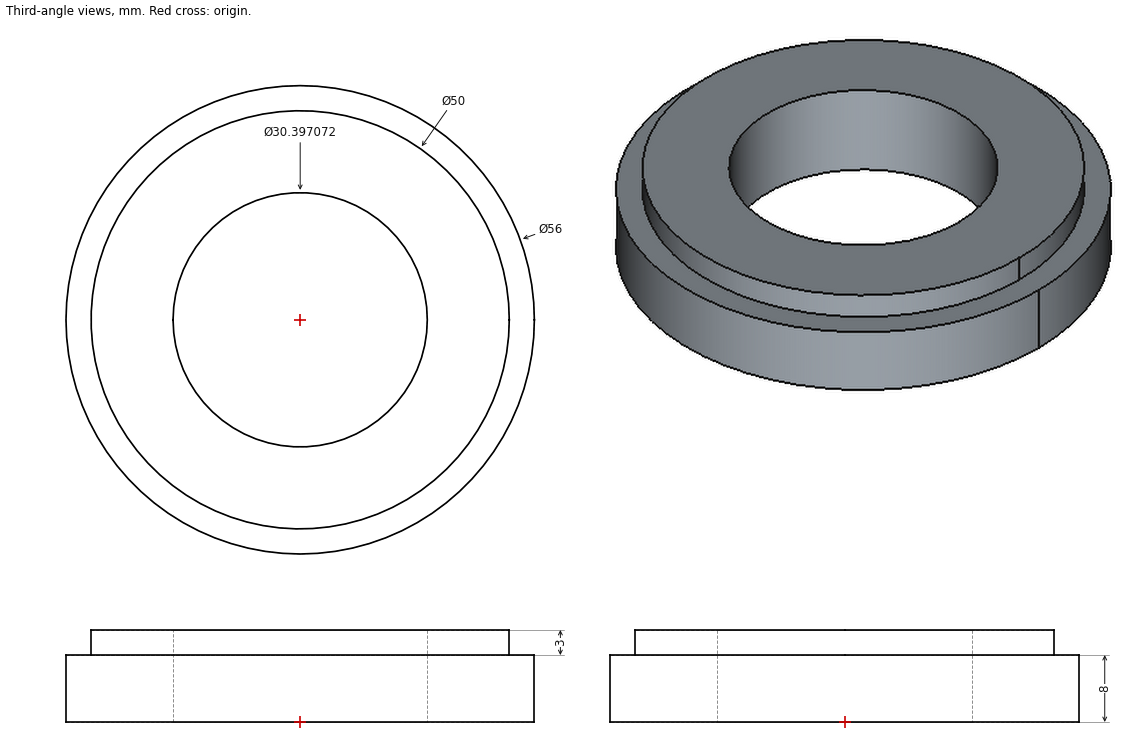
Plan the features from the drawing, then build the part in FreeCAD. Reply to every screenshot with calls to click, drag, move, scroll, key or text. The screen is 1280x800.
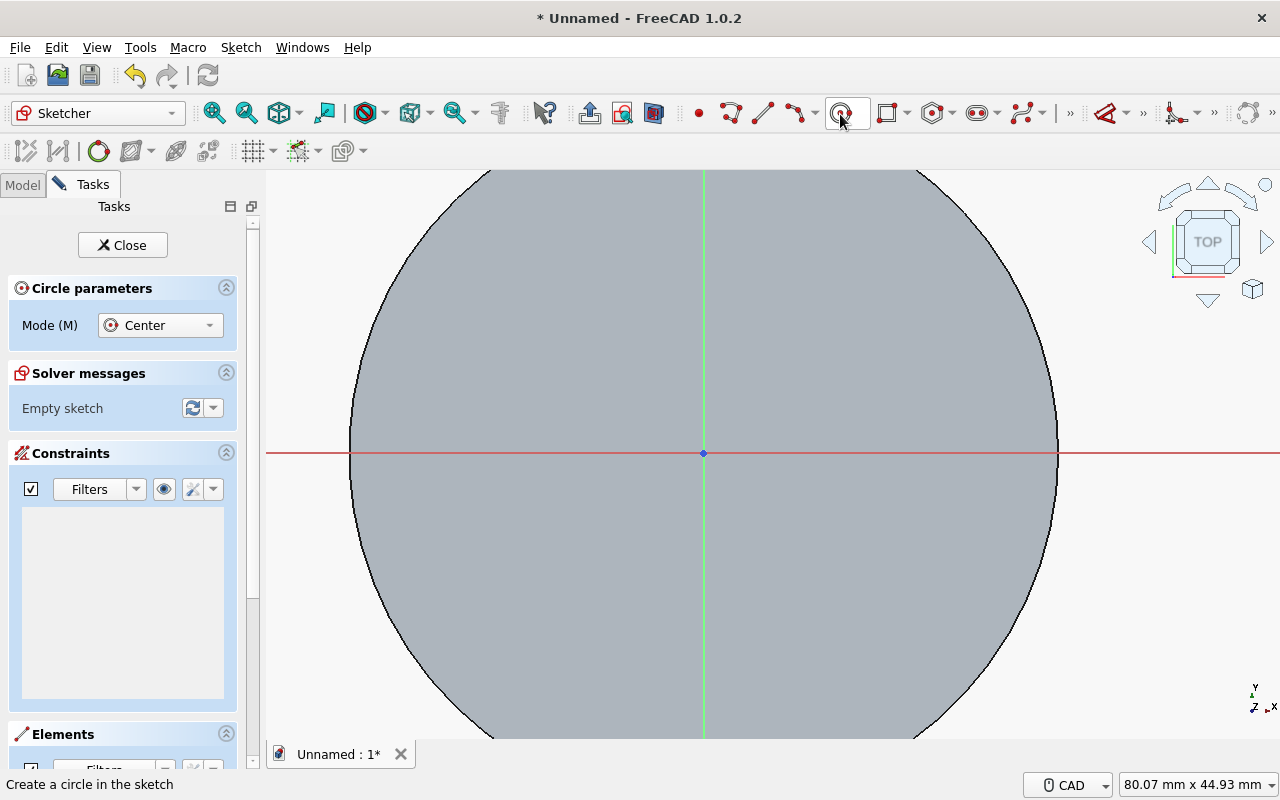
click(704, 453)
click(840, 317)
key(Escape)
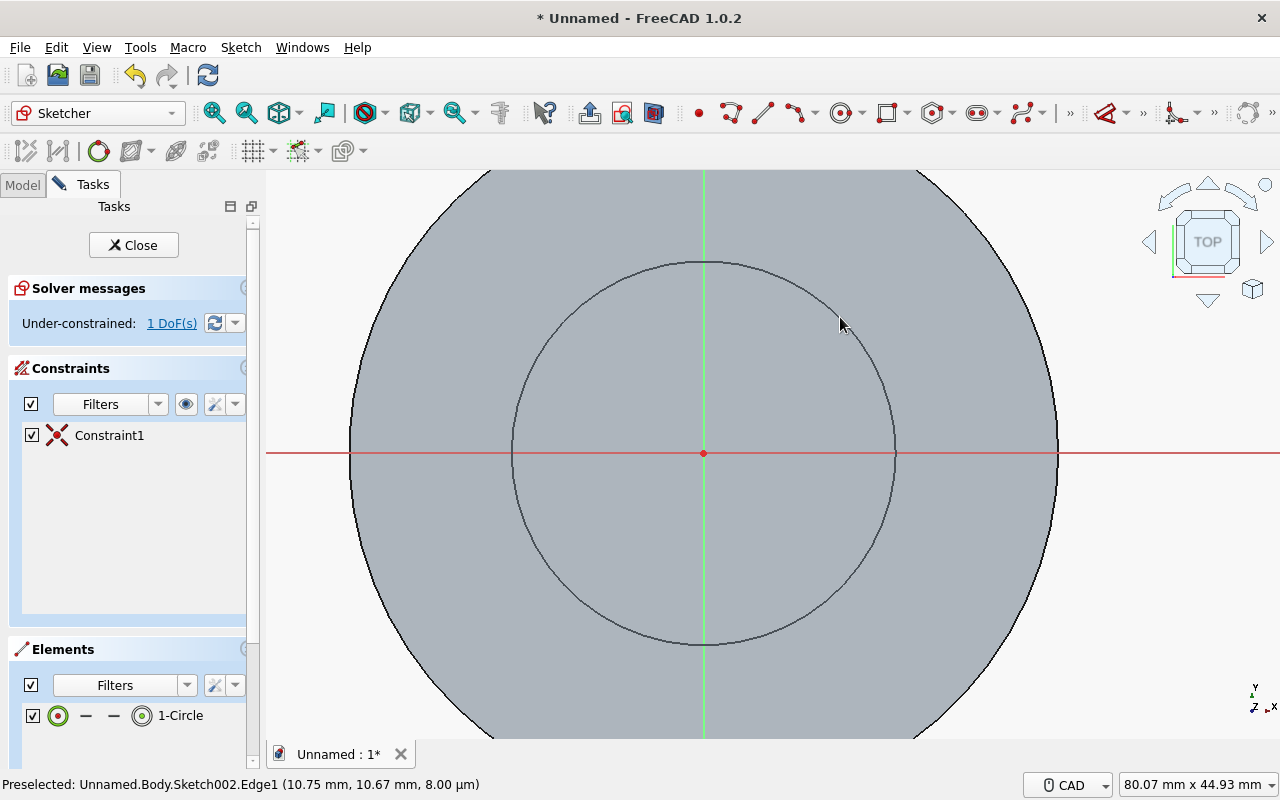
click(1106, 114)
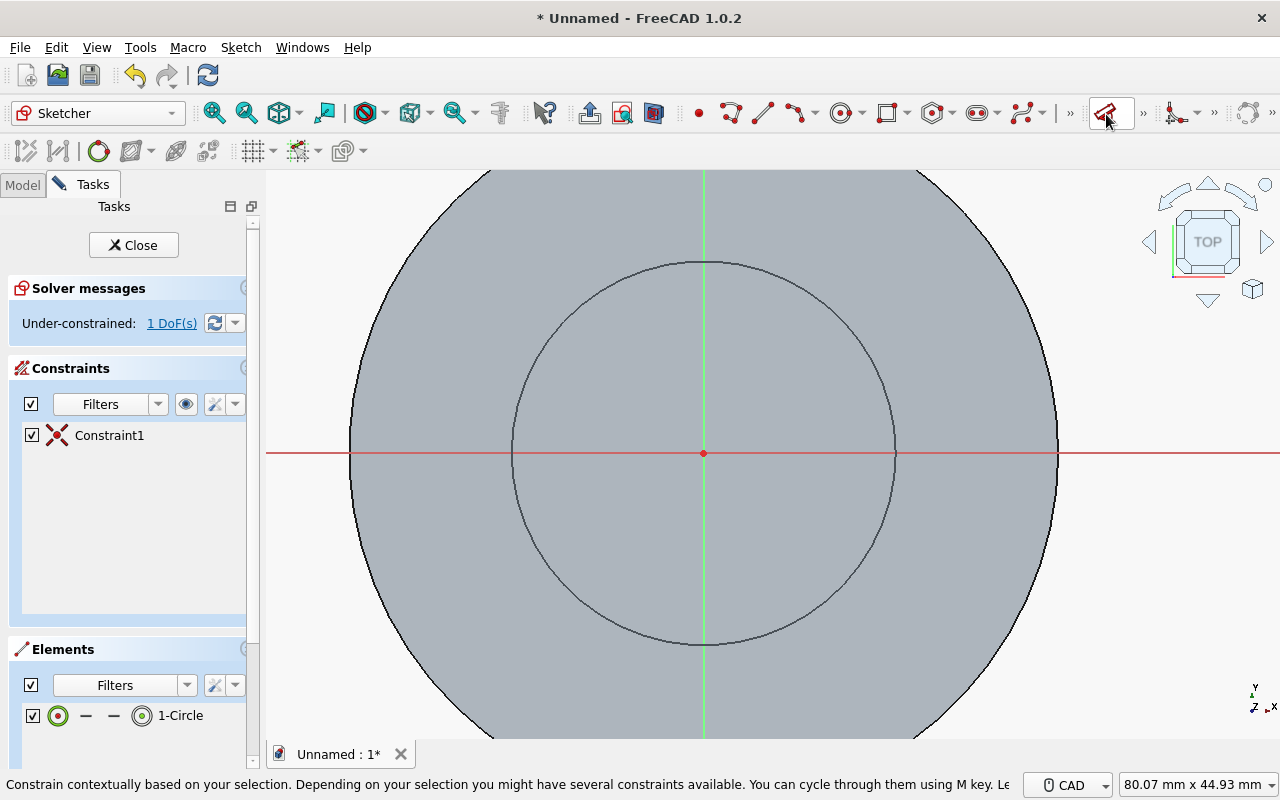
click(839, 317)
click(862, 294)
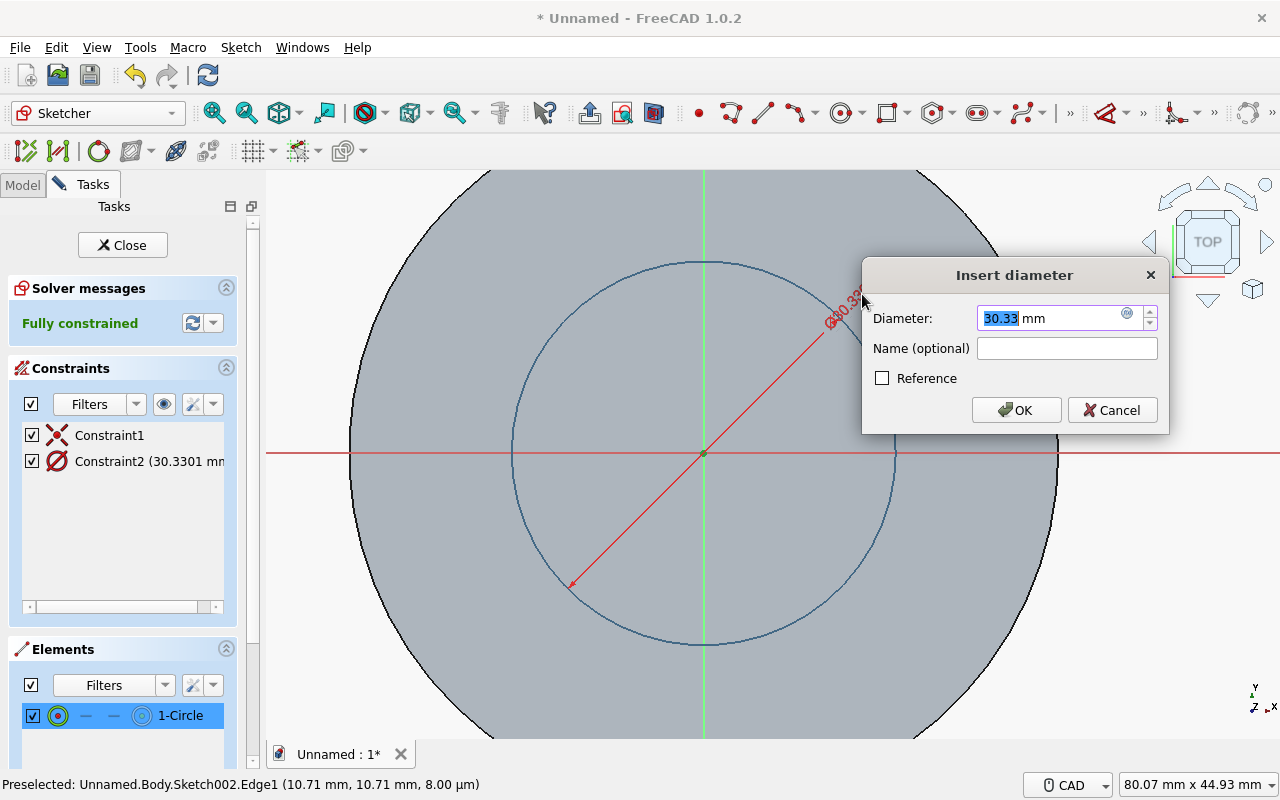
text(30.397072)
key(Return)
key(Escape)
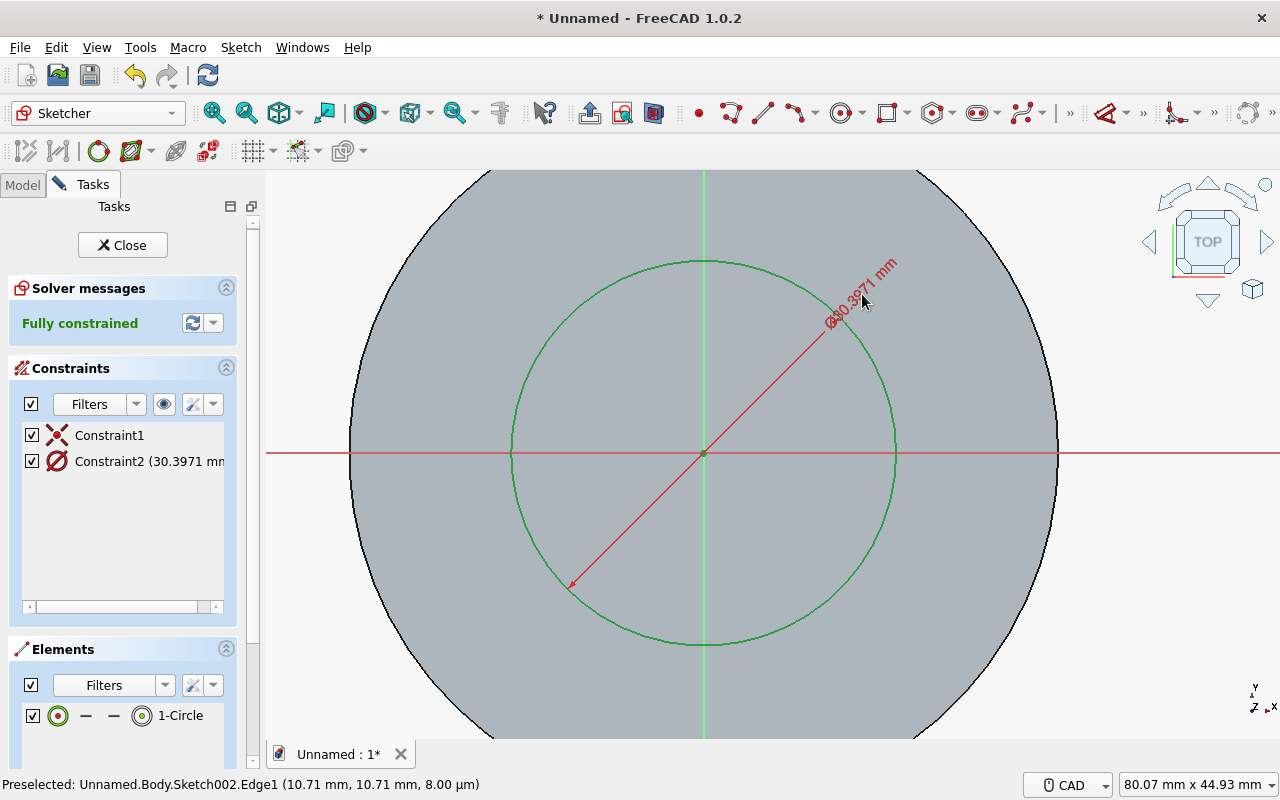
click(123, 245)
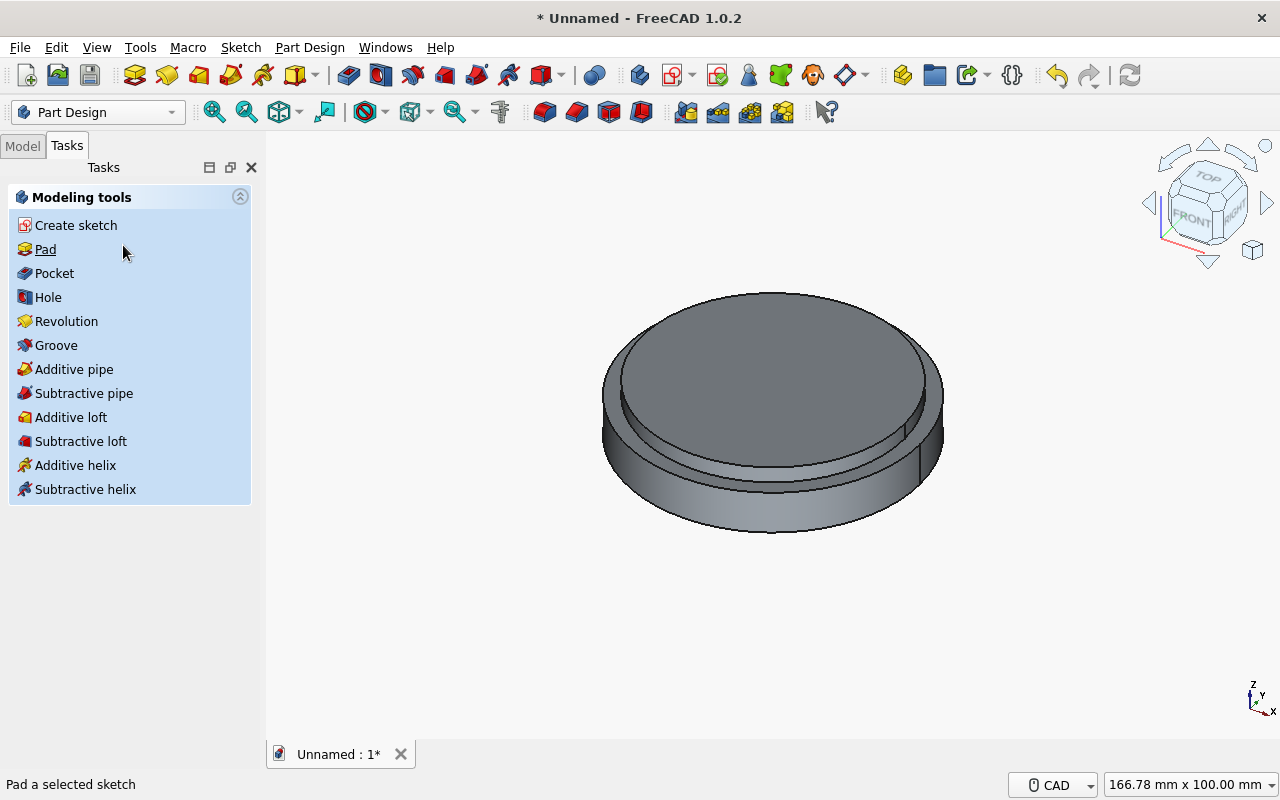
click(350, 76)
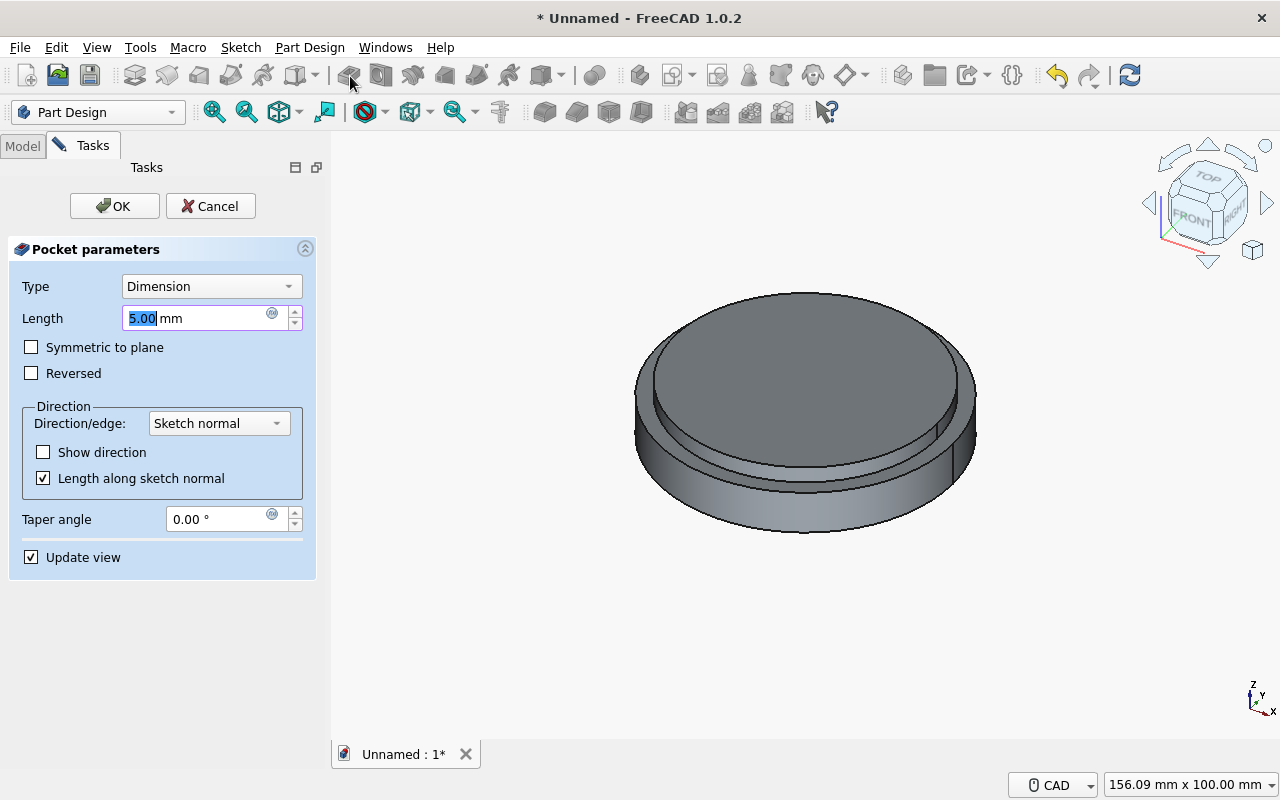
click(212, 286)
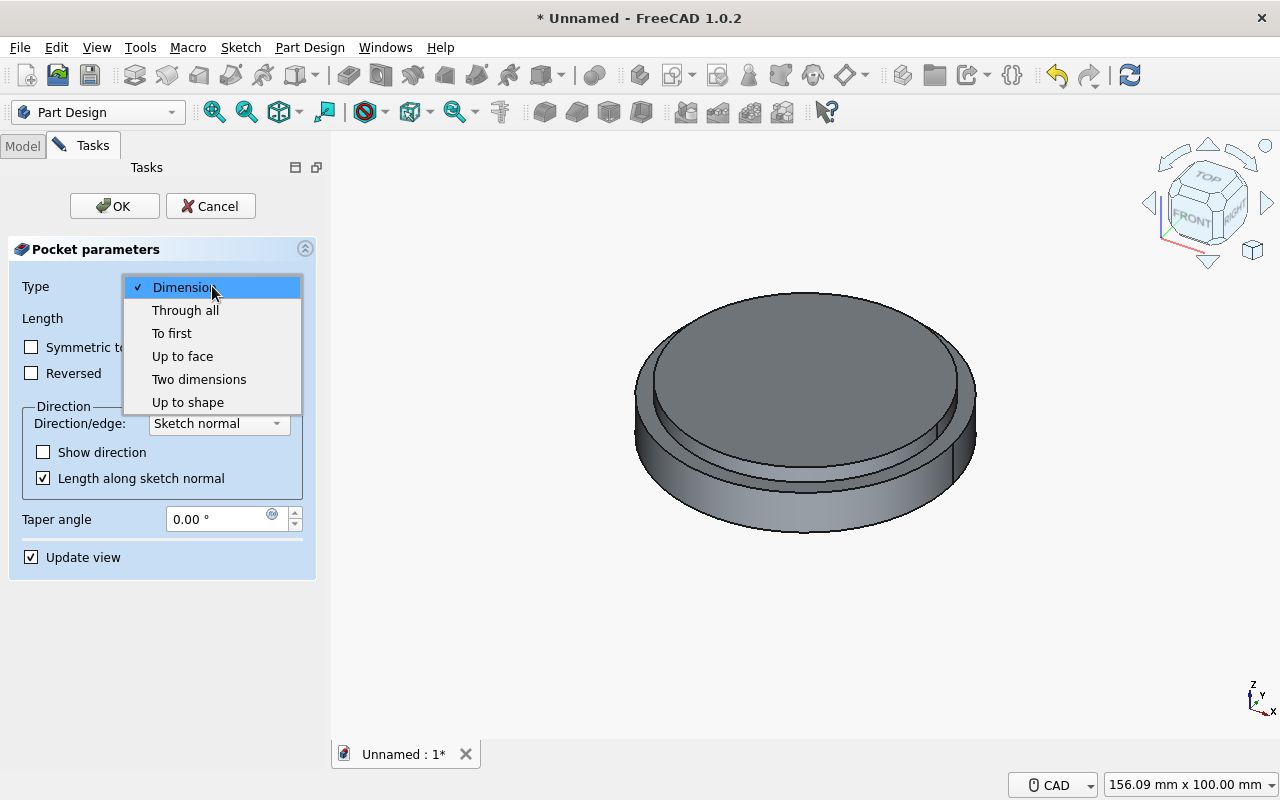
click(212, 310)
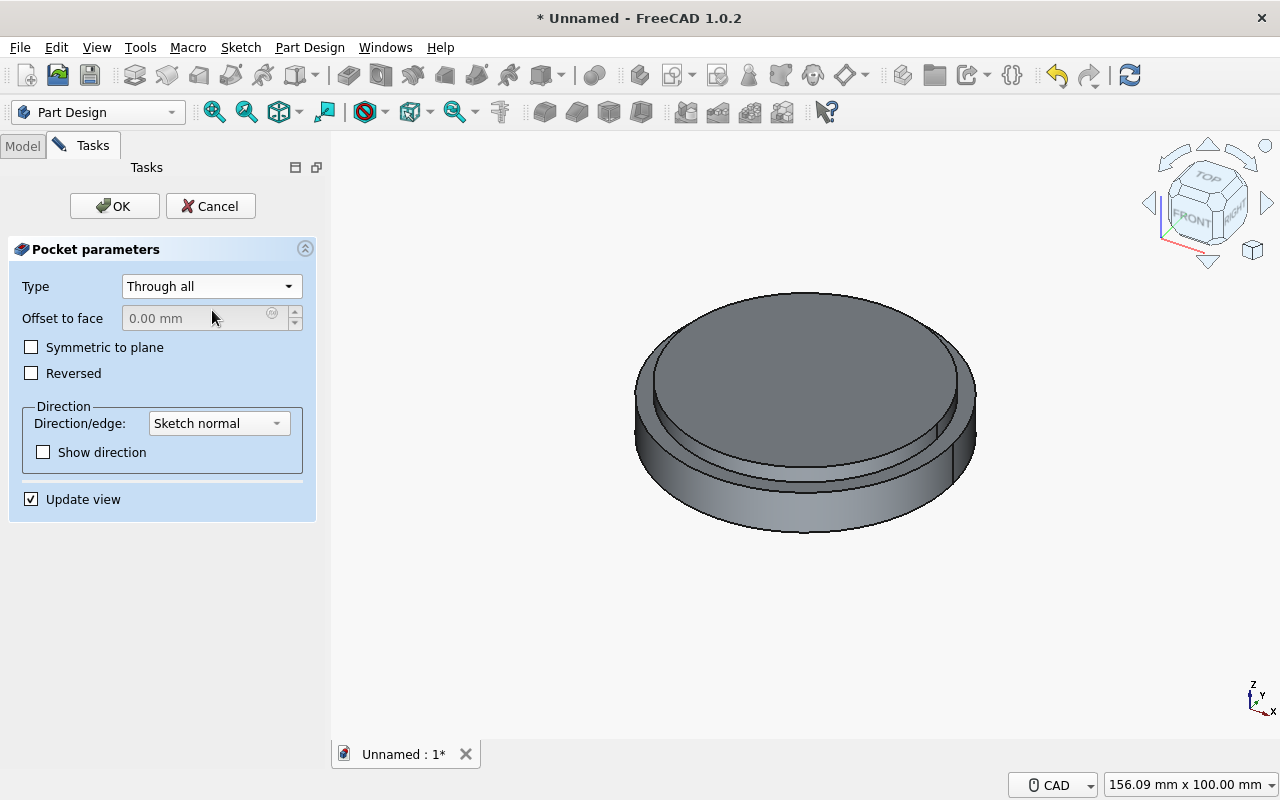
click(30, 373)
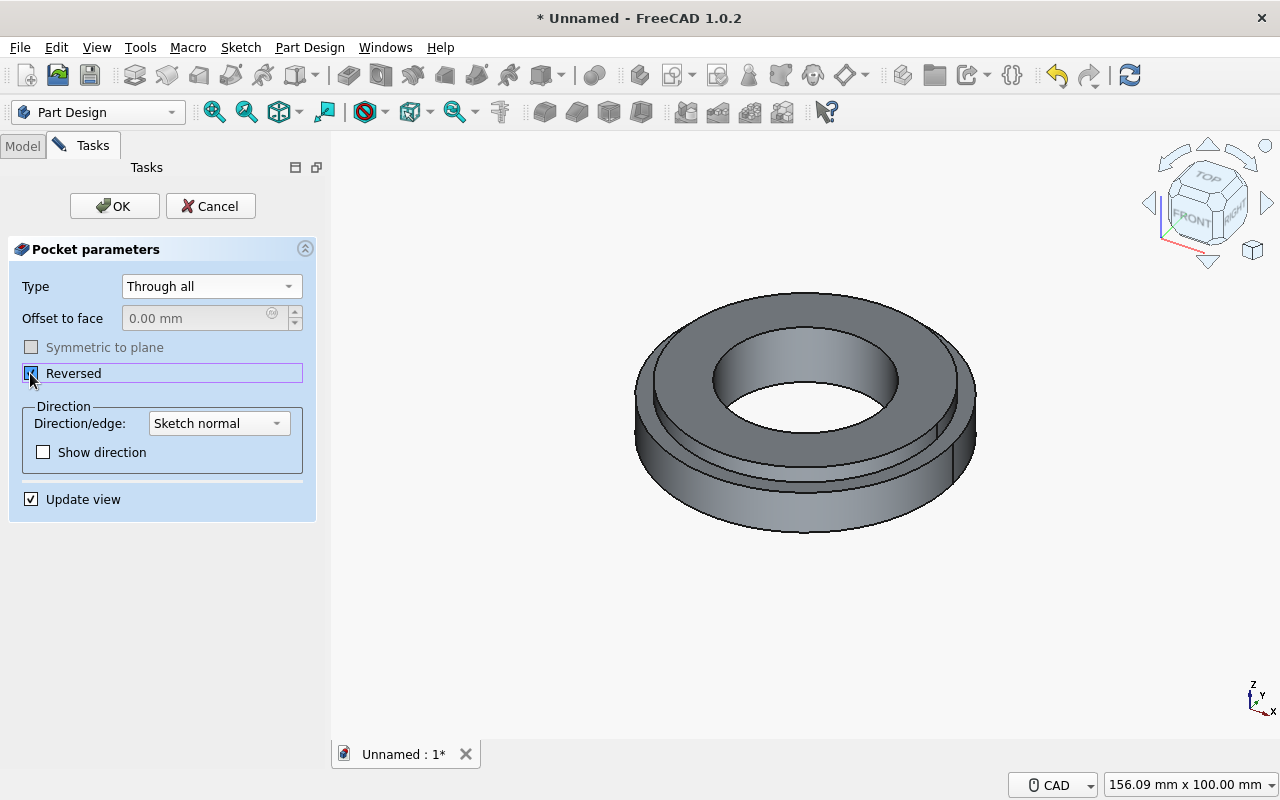
click(115, 206)